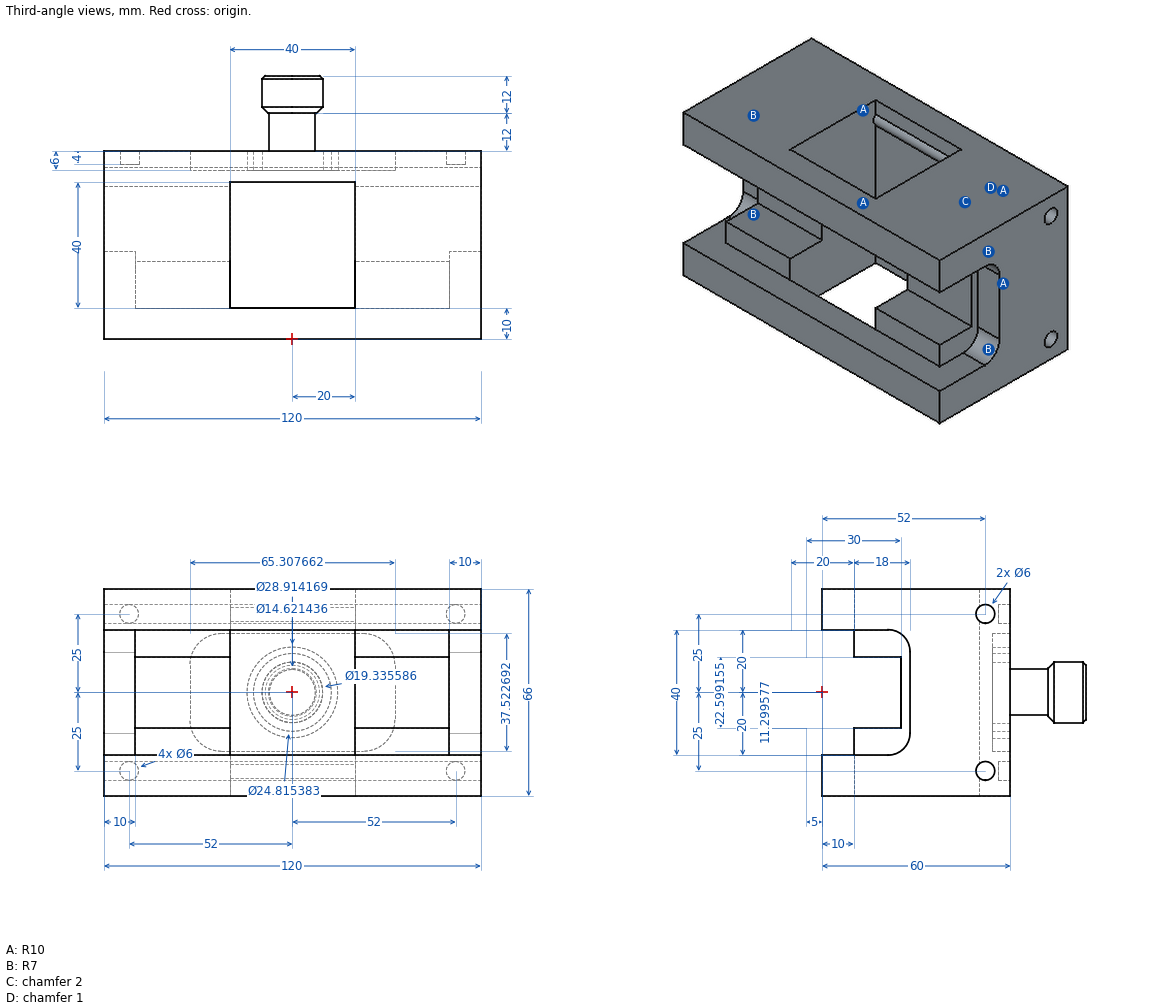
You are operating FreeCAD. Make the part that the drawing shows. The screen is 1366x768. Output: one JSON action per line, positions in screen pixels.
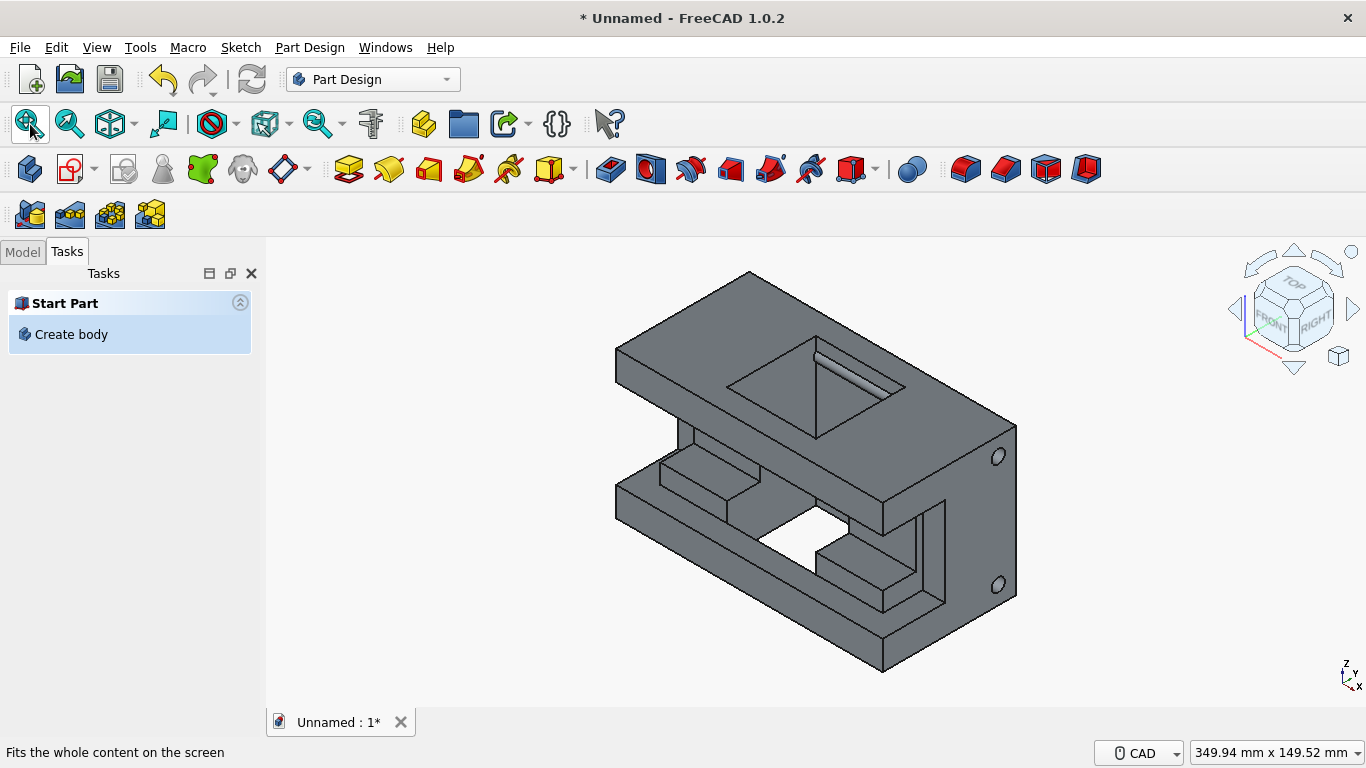
{"action": "scroll", "coordinate": [949, 526], "scroll_direction": "up", "scroll_amount": 4}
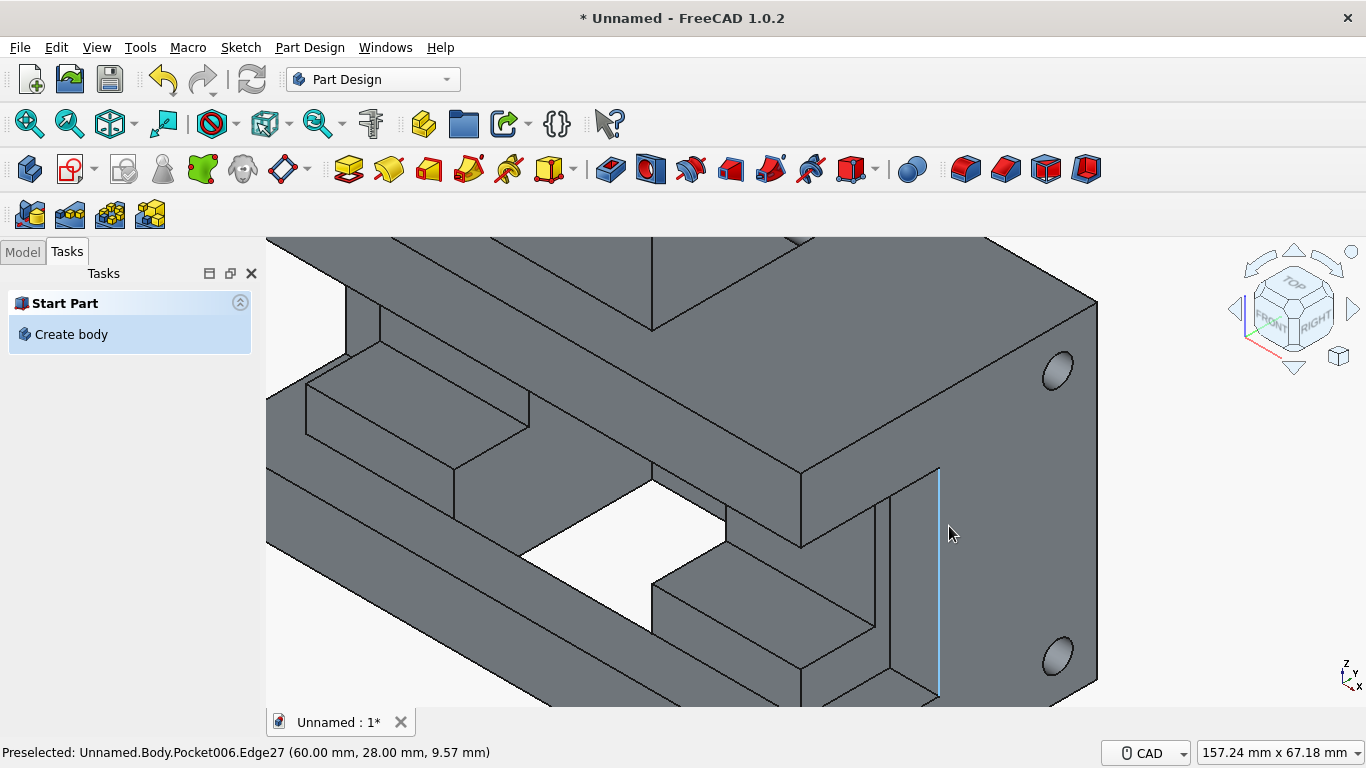
{"action": "left_click", "coordinate": [30, 124]}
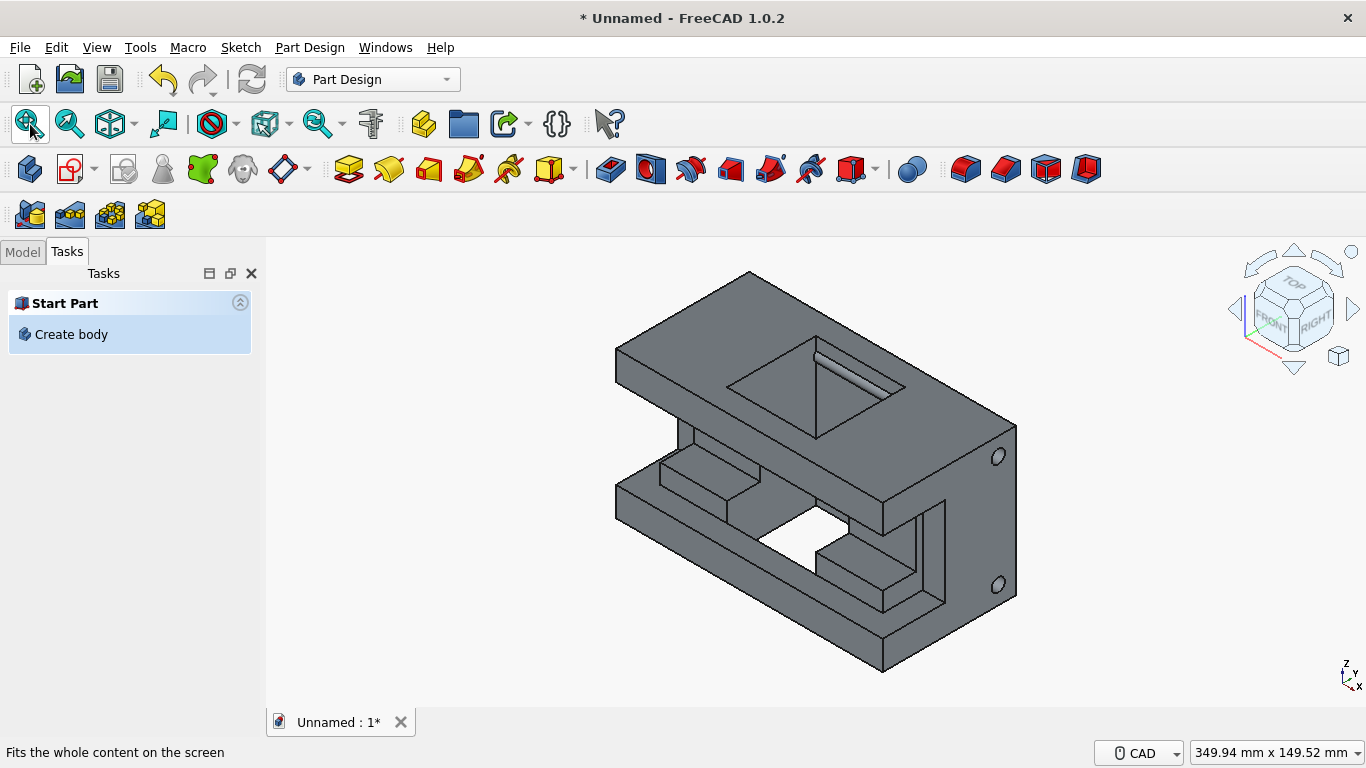
{"action": "key", "text": "2"}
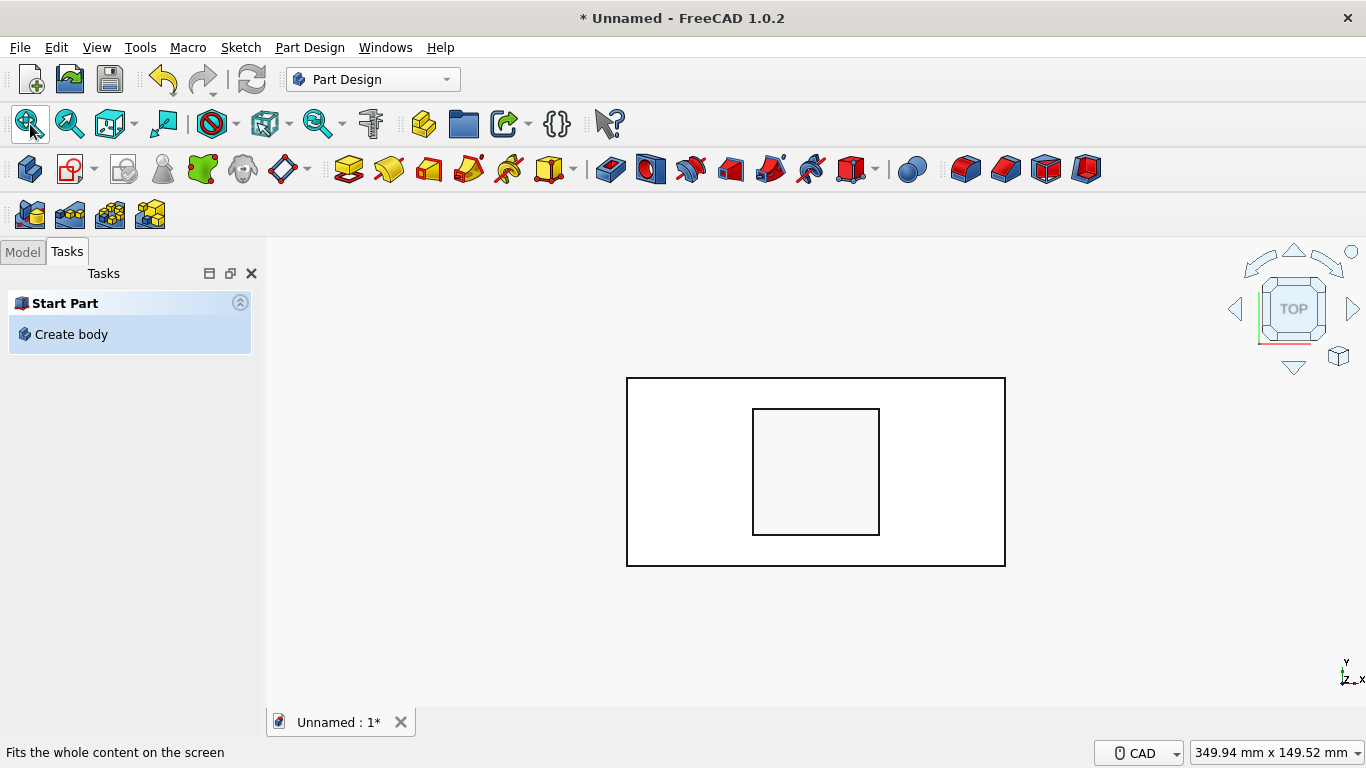
{"action": "left_click", "coordinate": [30, 124]}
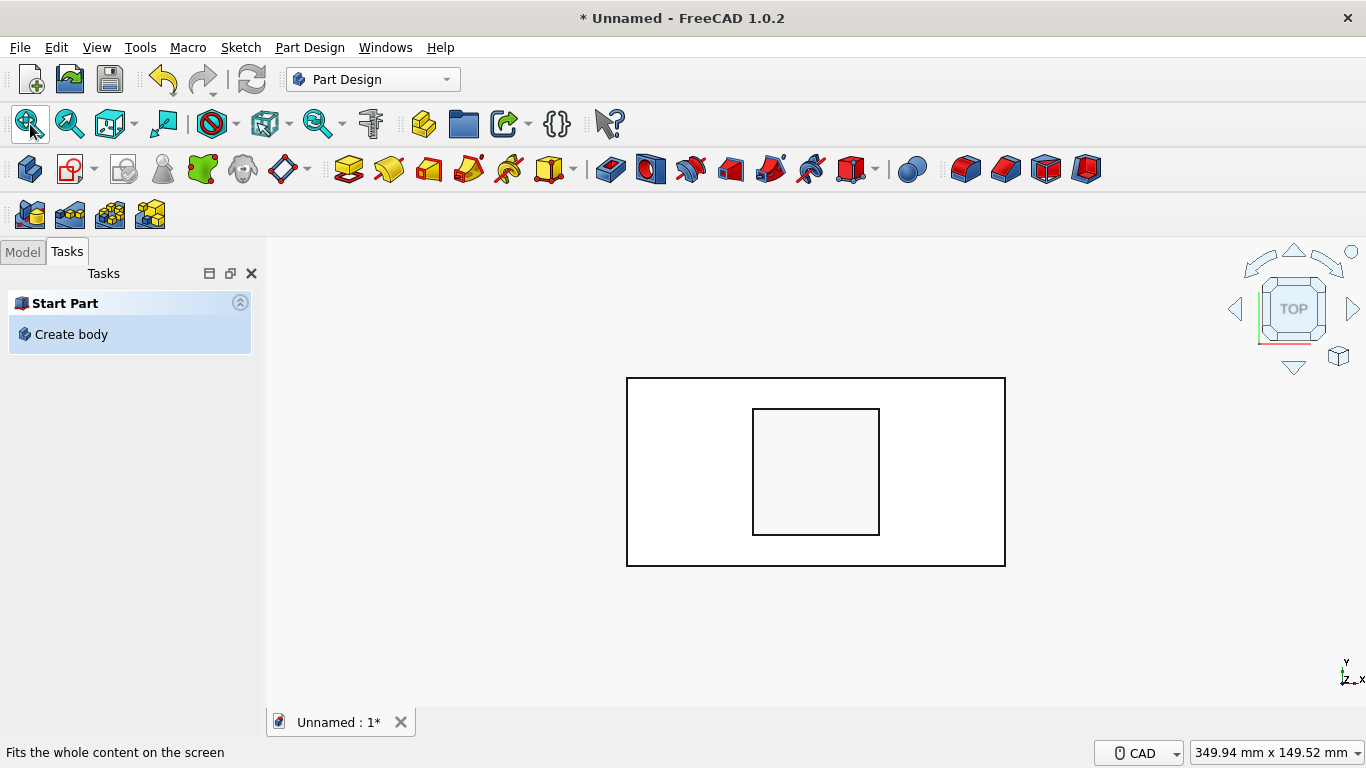
{"action": "scroll", "coordinate": [919, 386], "scroll_direction": "up", "scroll_amount": 4}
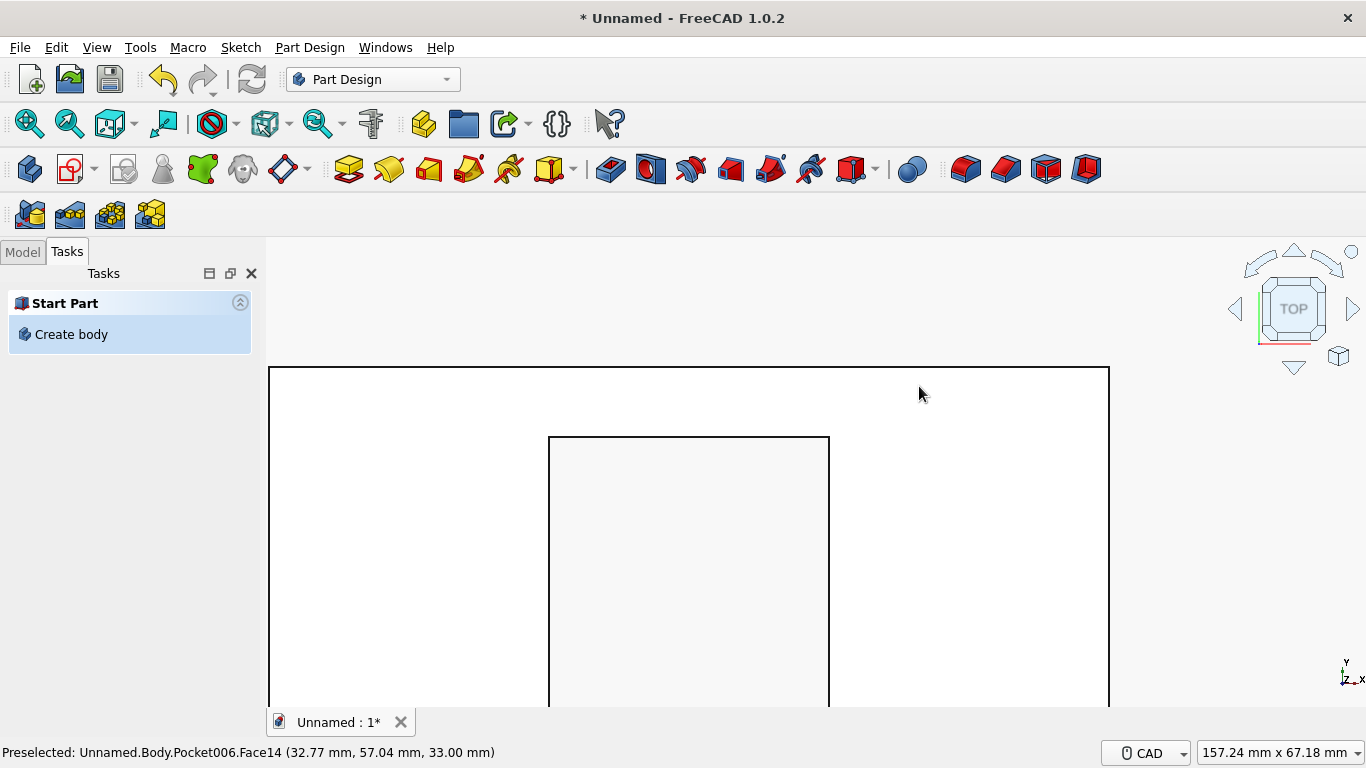
{"action": "left_click", "coordinate": [30, 124]}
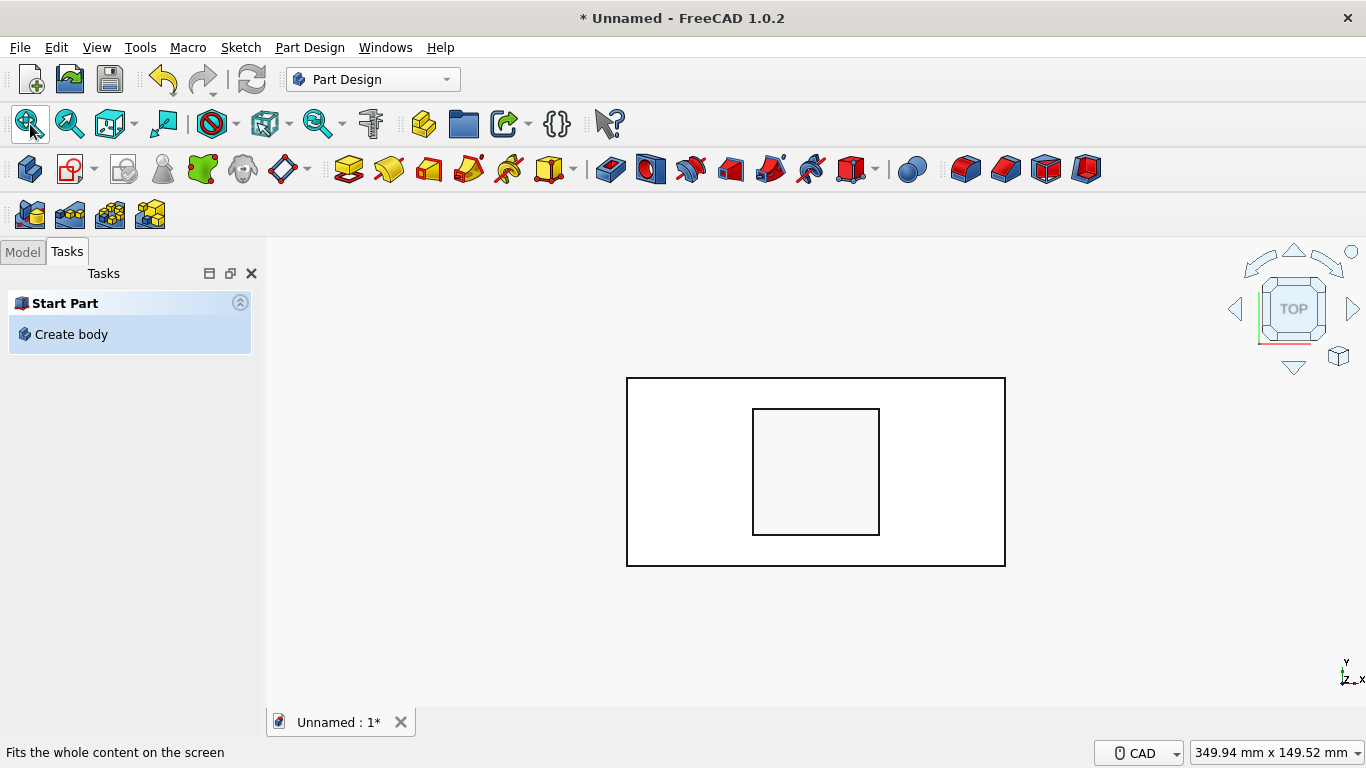
{"action": "key", "text": "1"}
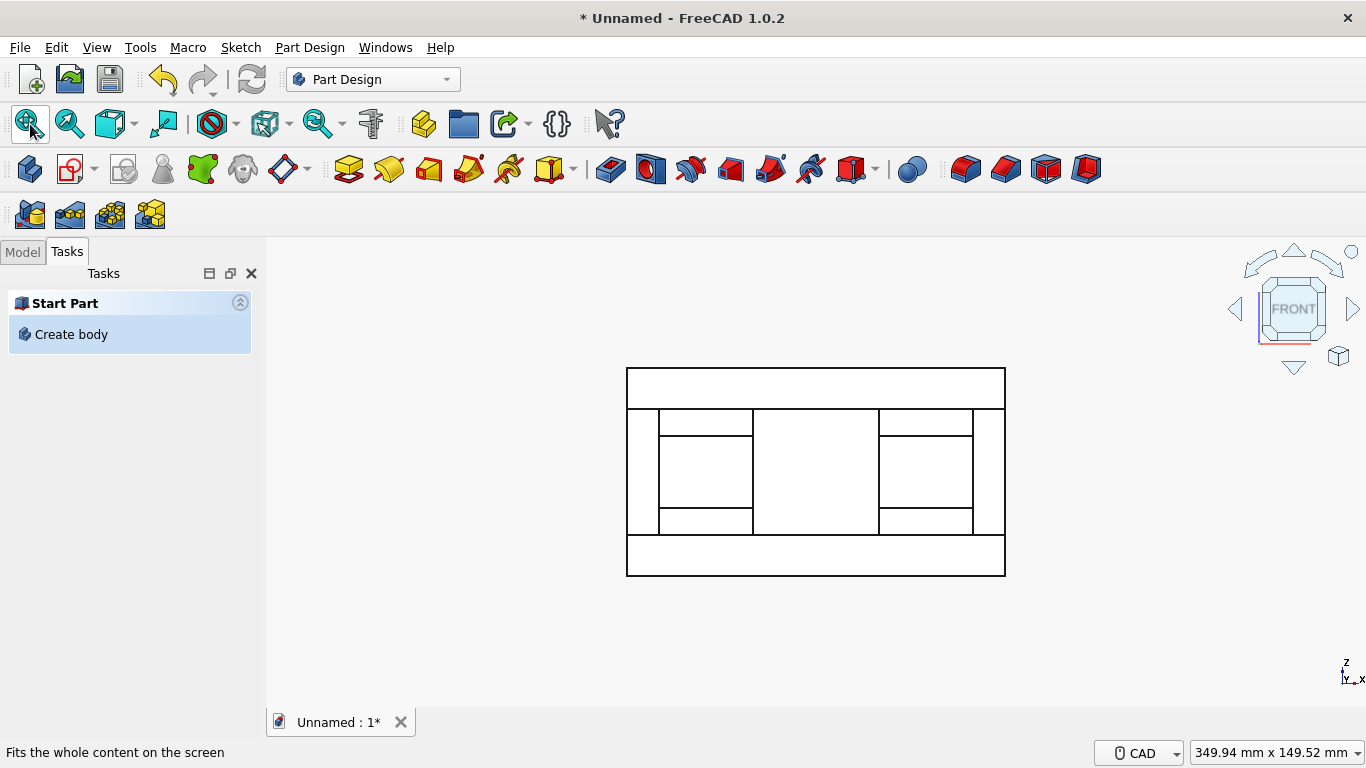
{"action": "left_click", "coordinate": [30, 124]}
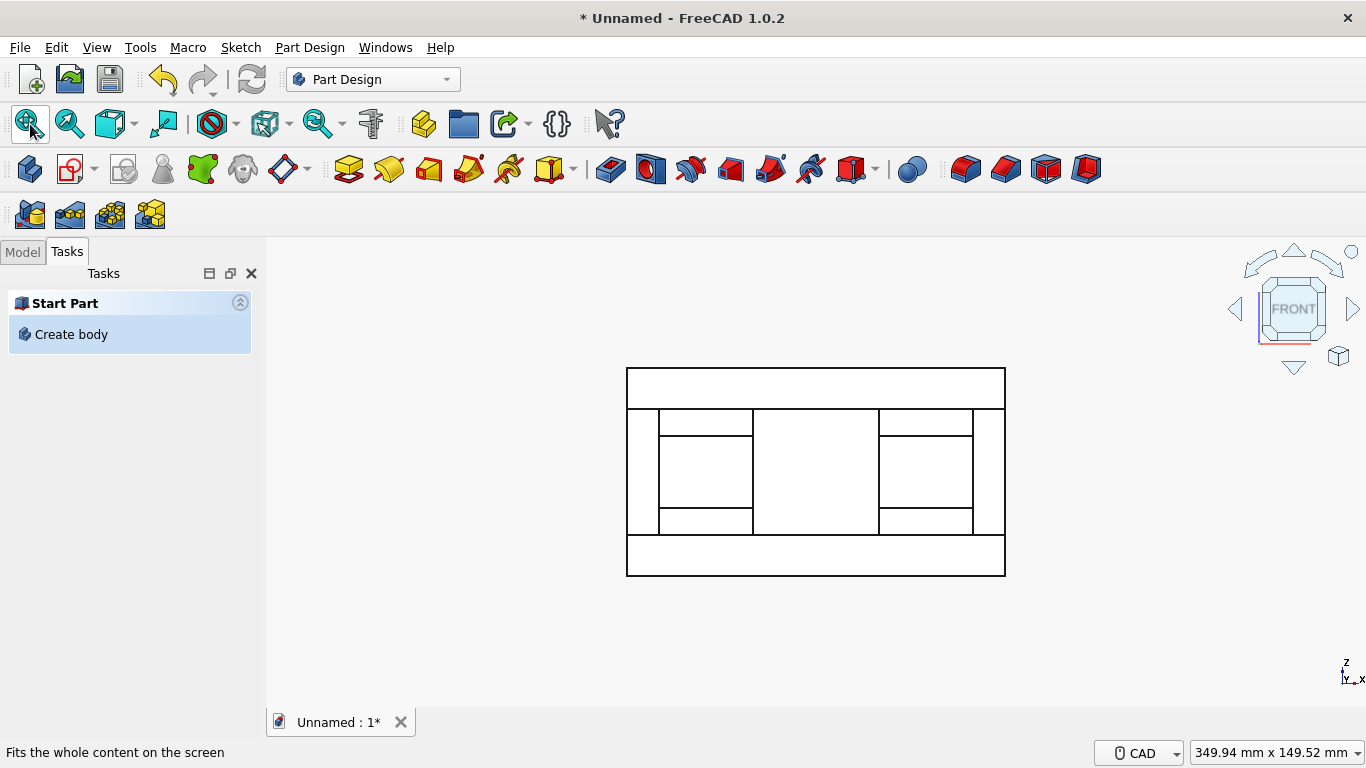
{"action": "scroll", "coordinate": [919, 530], "scroll_direction": "up", "scroll_amount": 4}